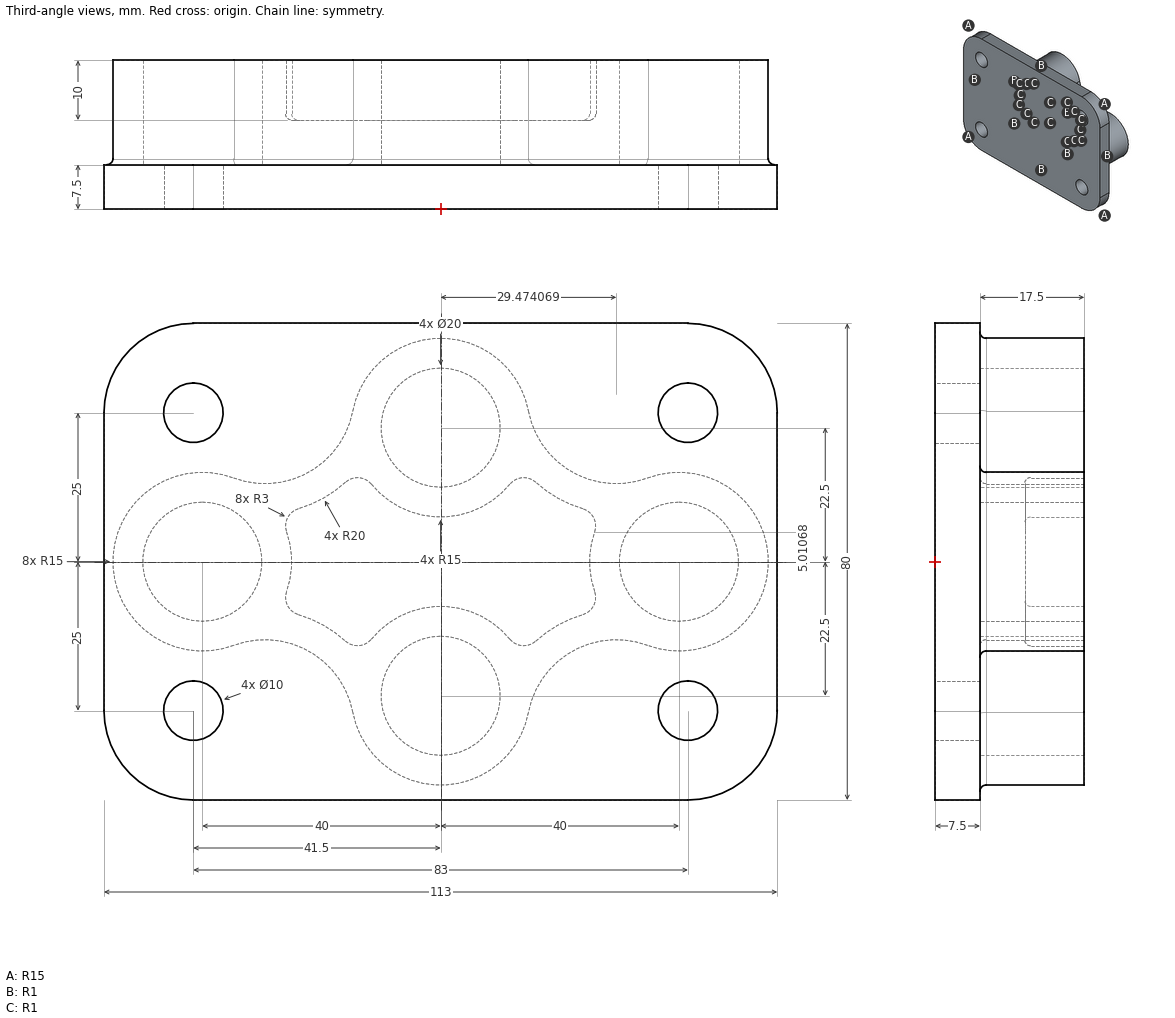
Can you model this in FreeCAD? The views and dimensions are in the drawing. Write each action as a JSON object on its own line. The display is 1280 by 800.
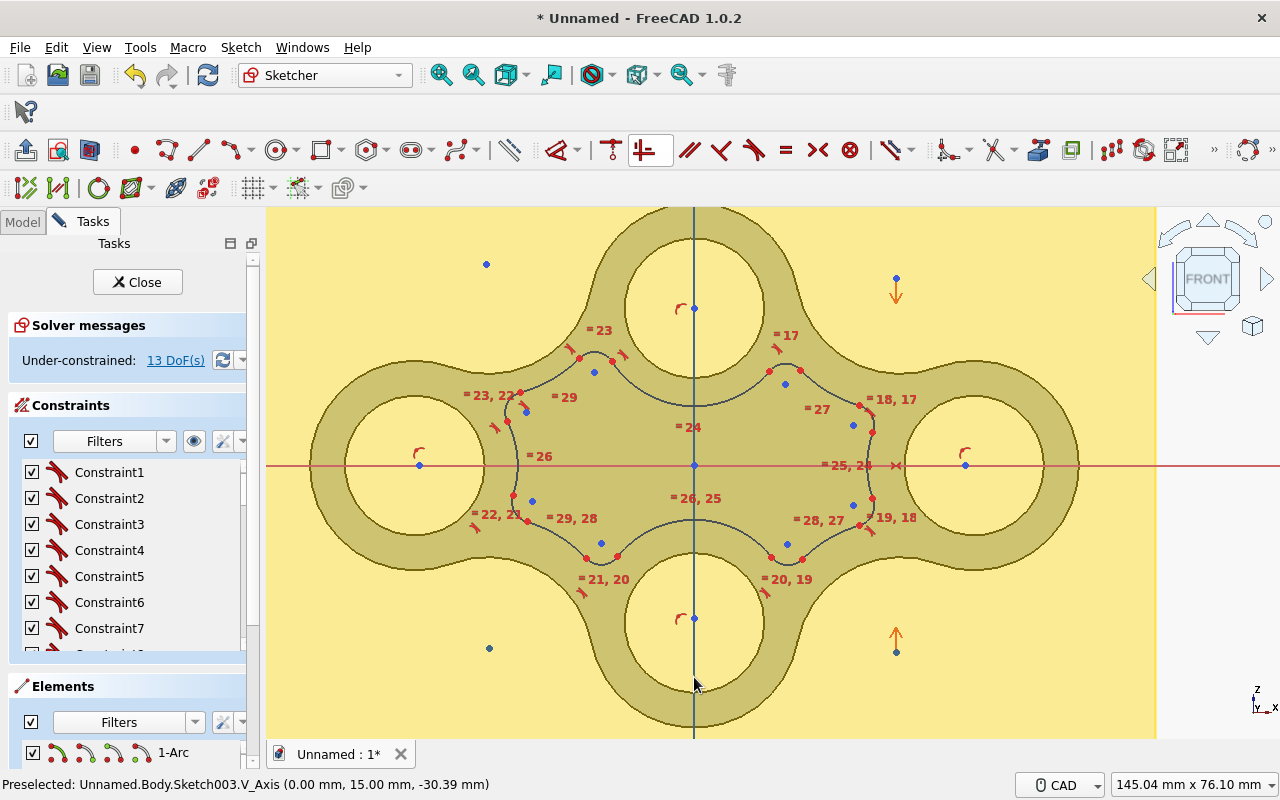
{"action": "key", "text": "s"}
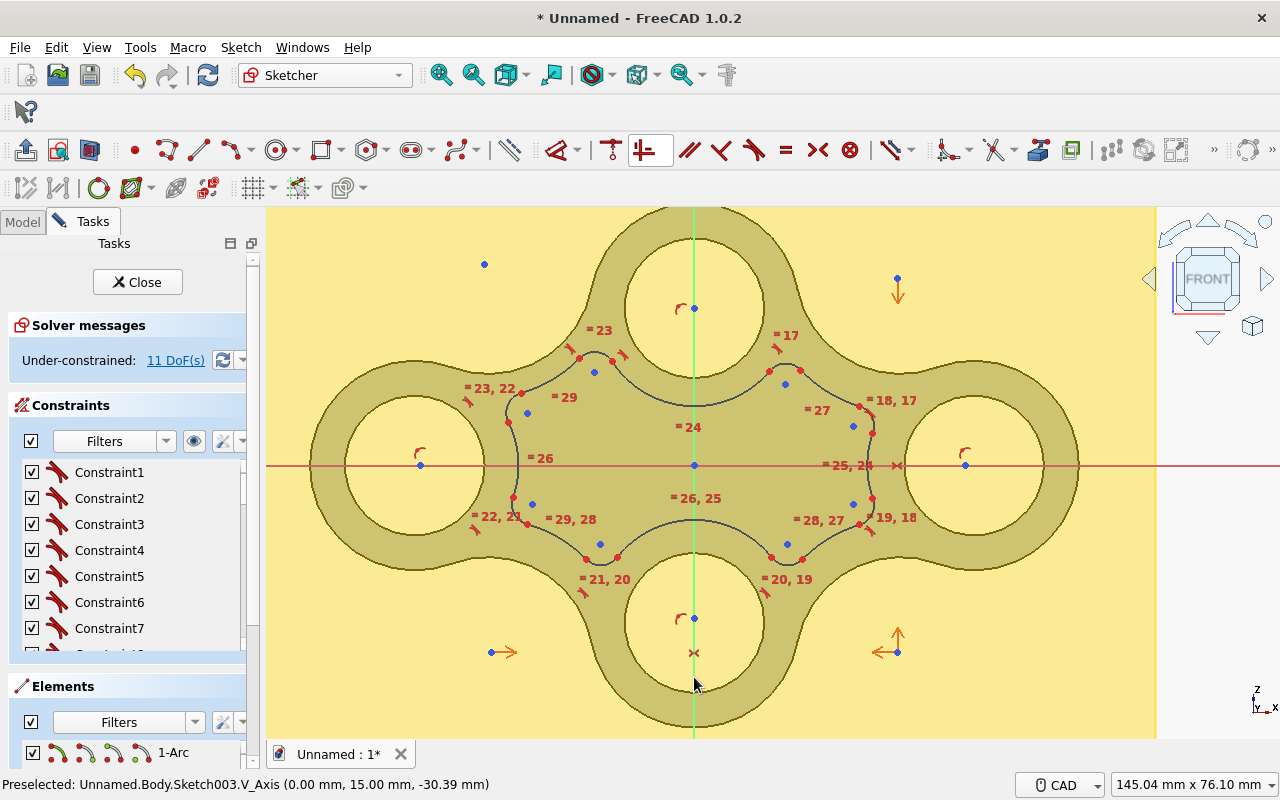
{"action": "left_click", "coordinate": [853, 426]}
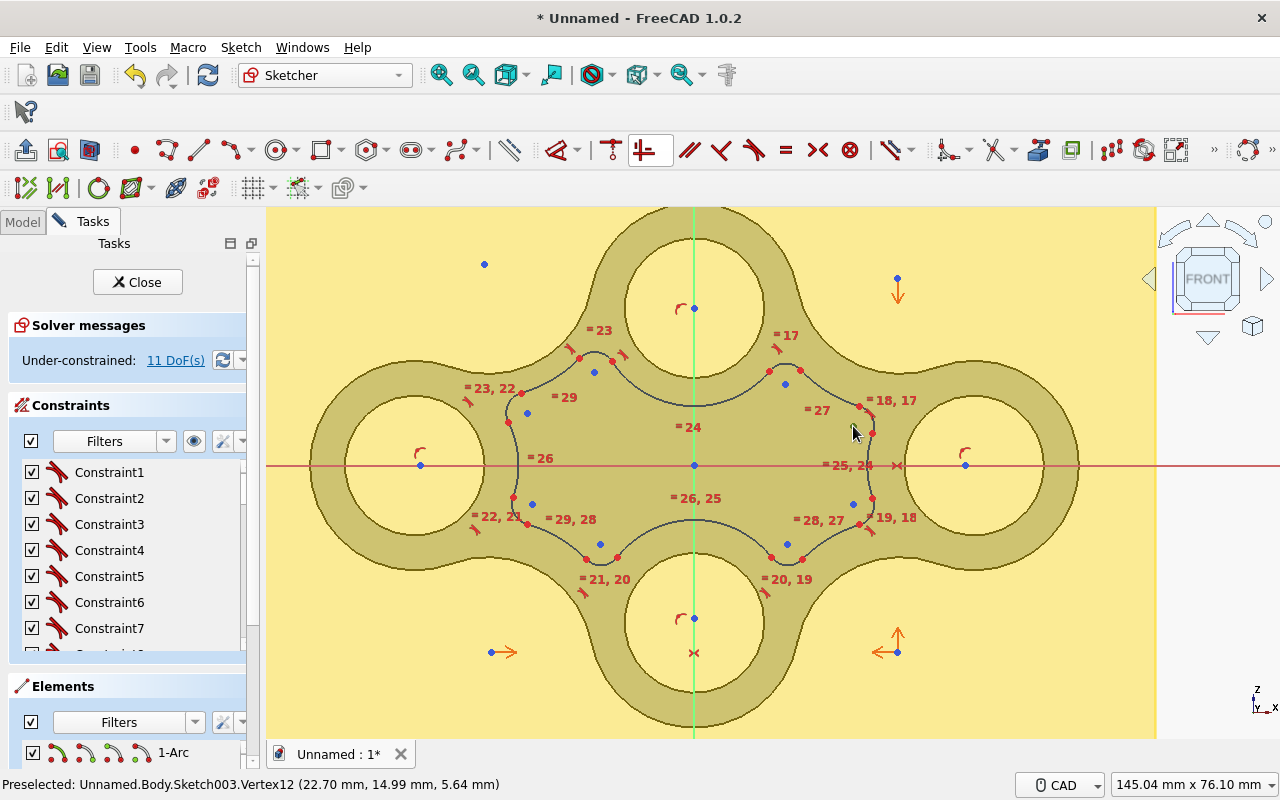
{"action": "left_click", "coordinate": [527, 413]}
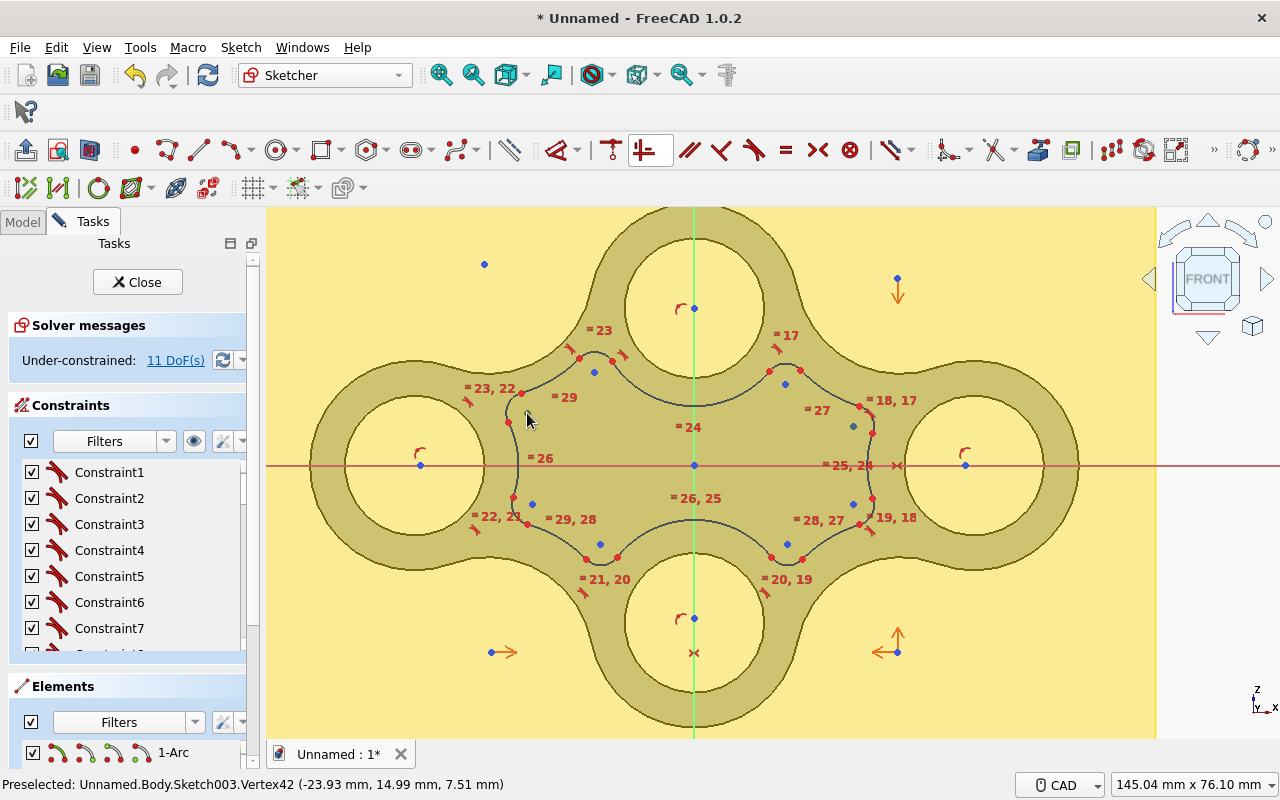
{"action": "left_click", "coordinate": [694, 677]}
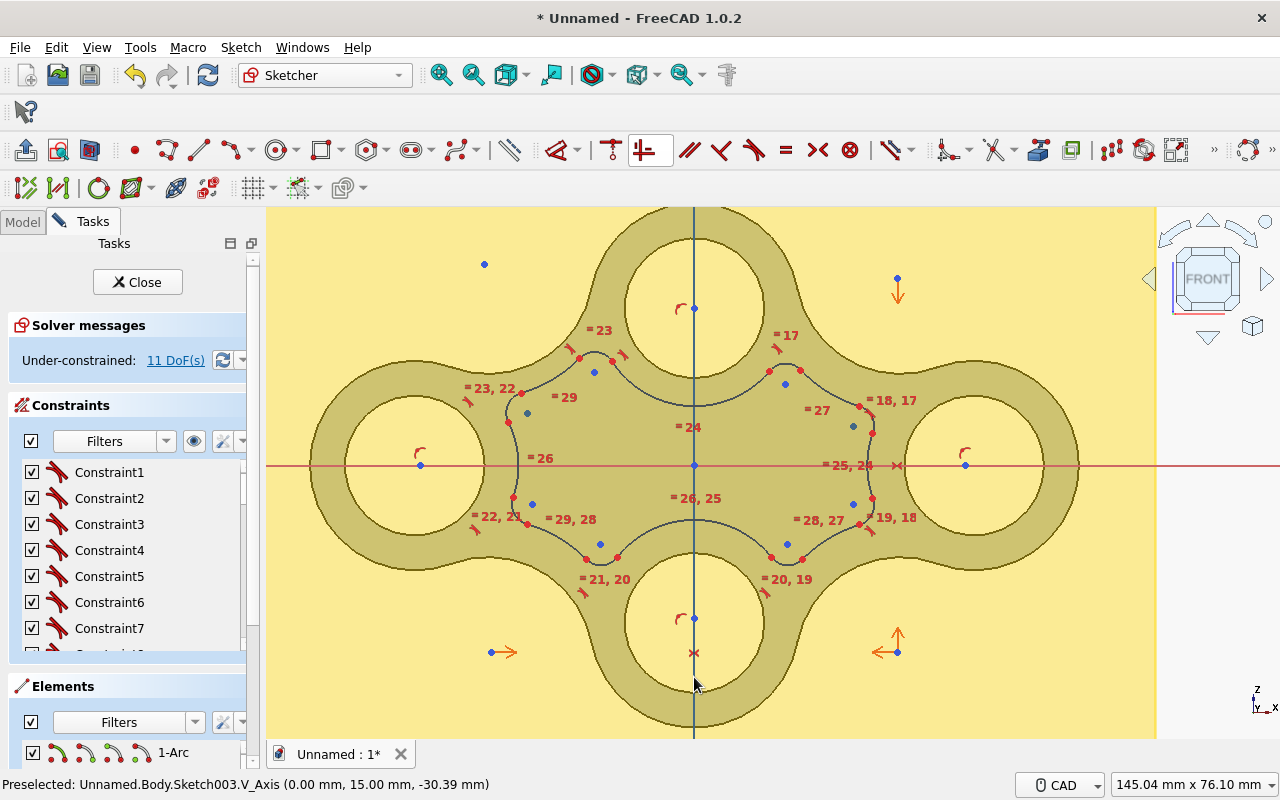
{"action": "key", "text": "s"}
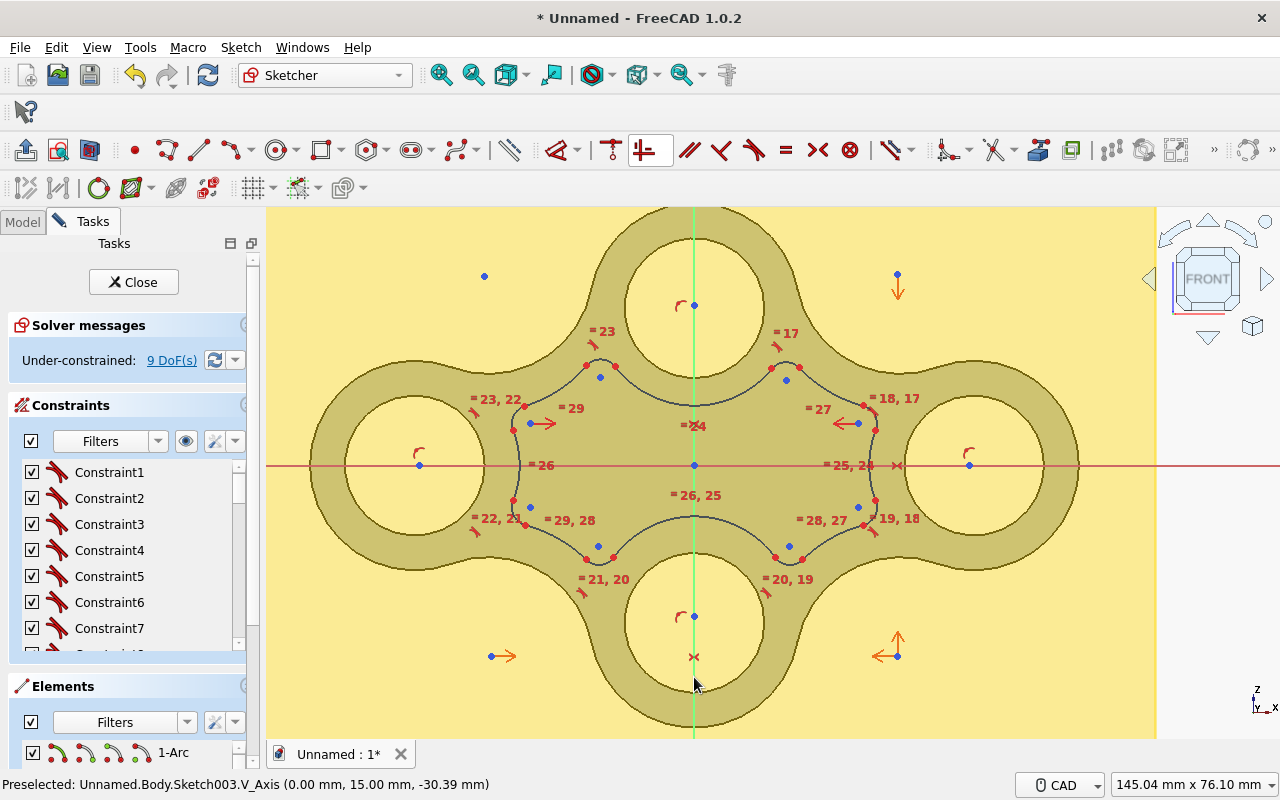
{"action": "left_click", "coordinate": [599, 547]}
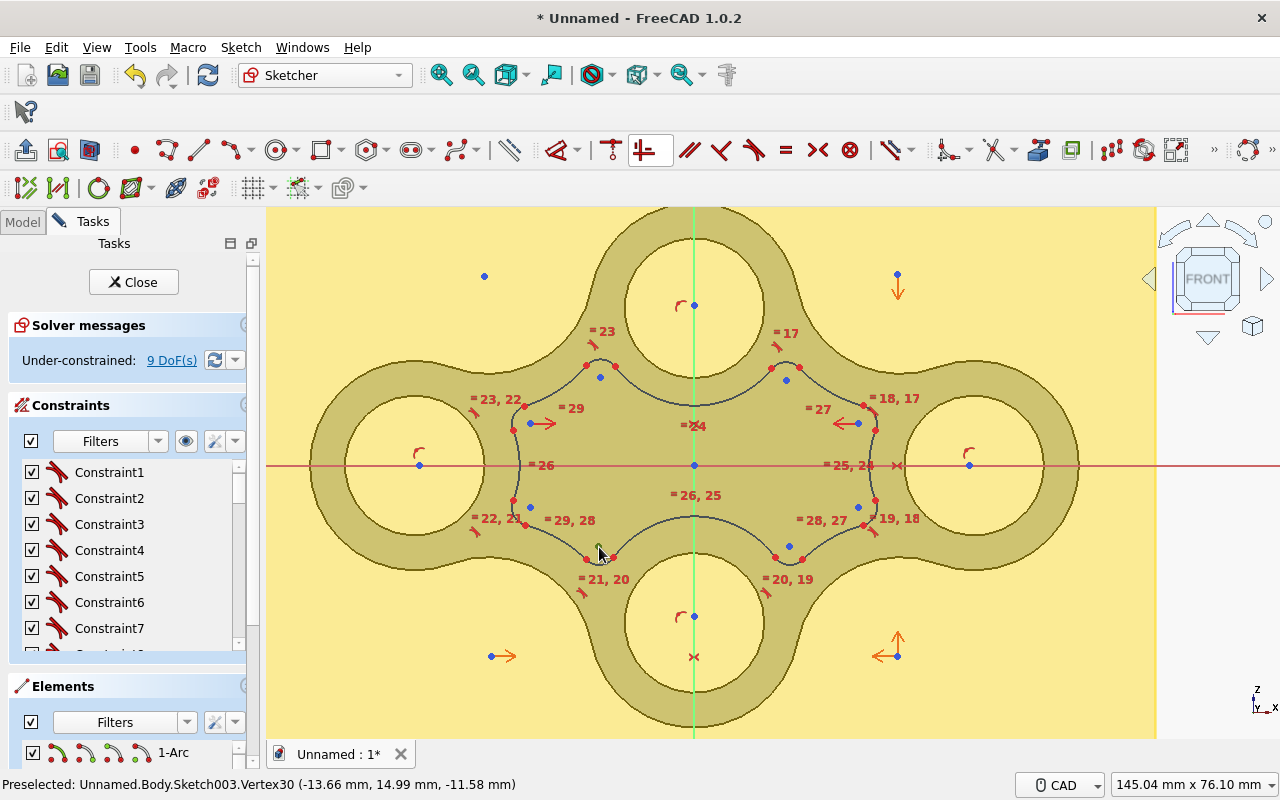
{"action": "left_click", "coordinate": [601, 378]}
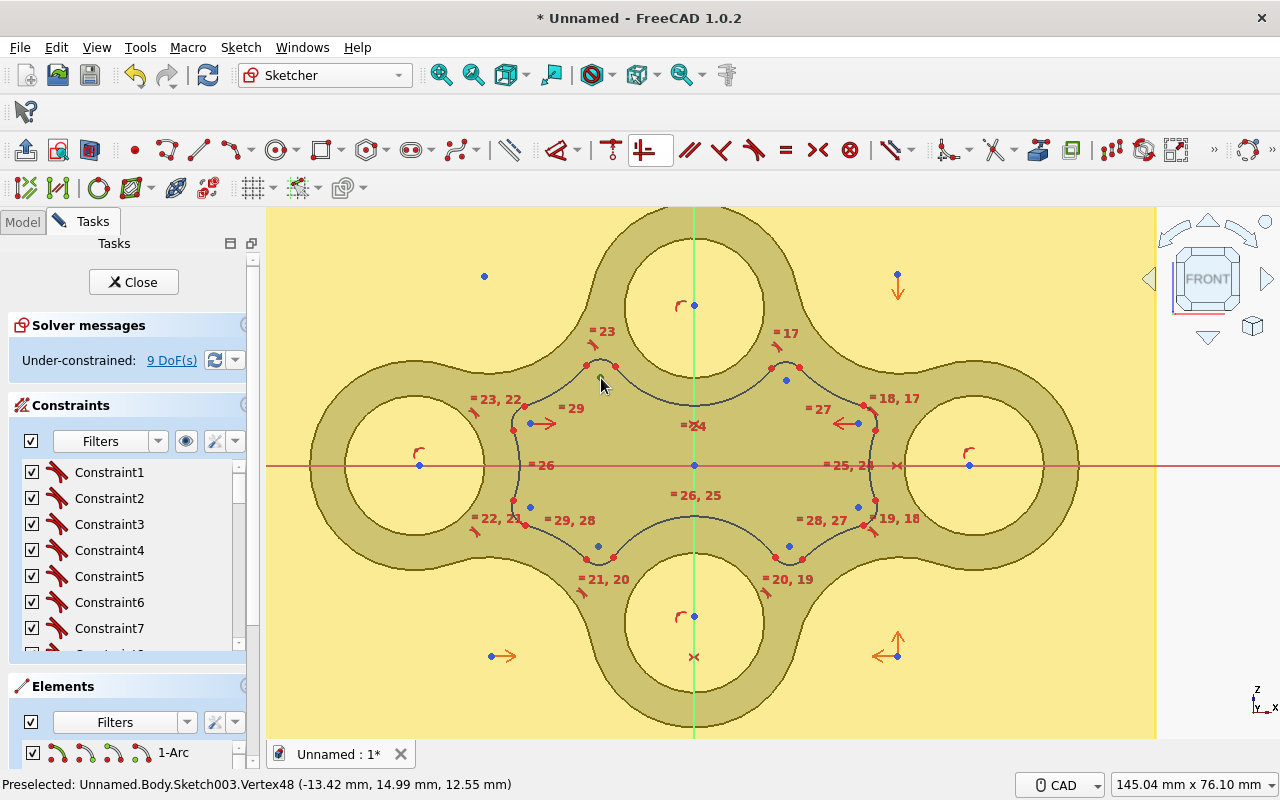
{"action": "left_click", "coordinate": [353, 466]}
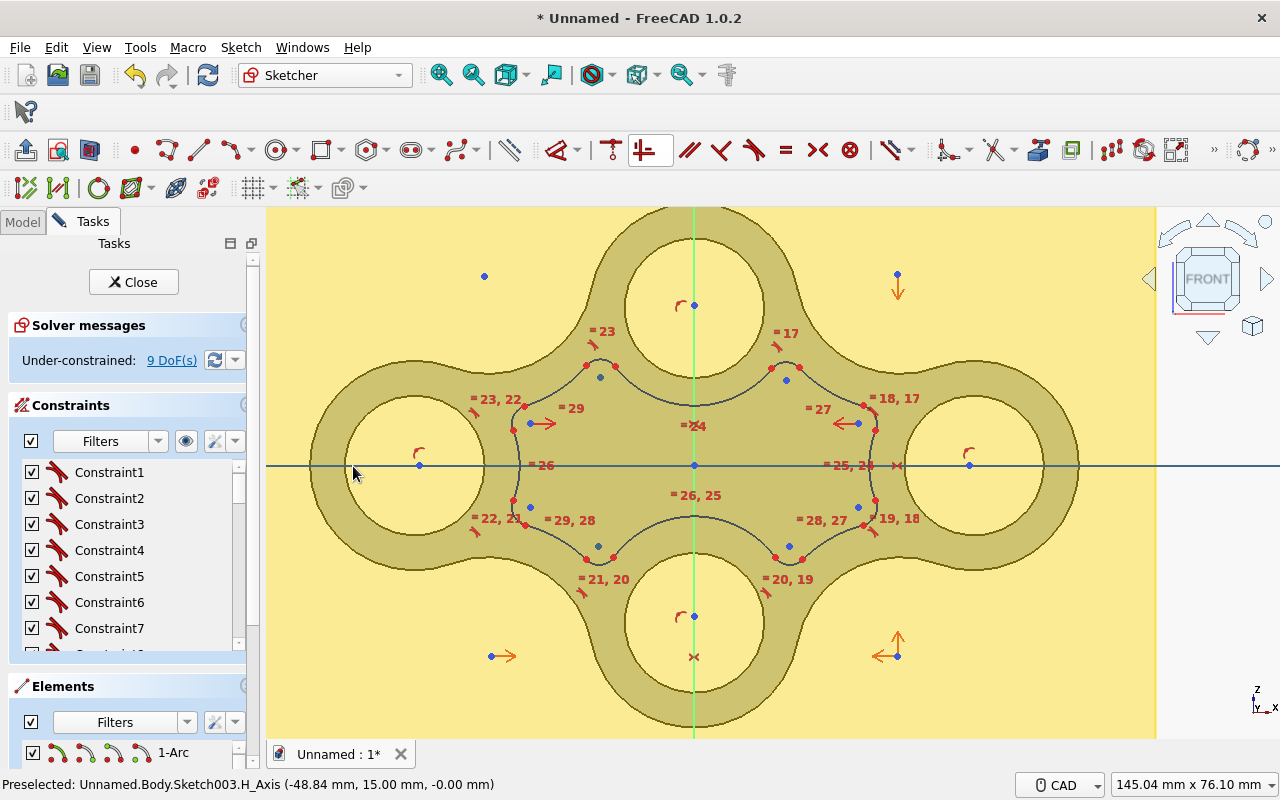
{"action": "key", "text": "s"}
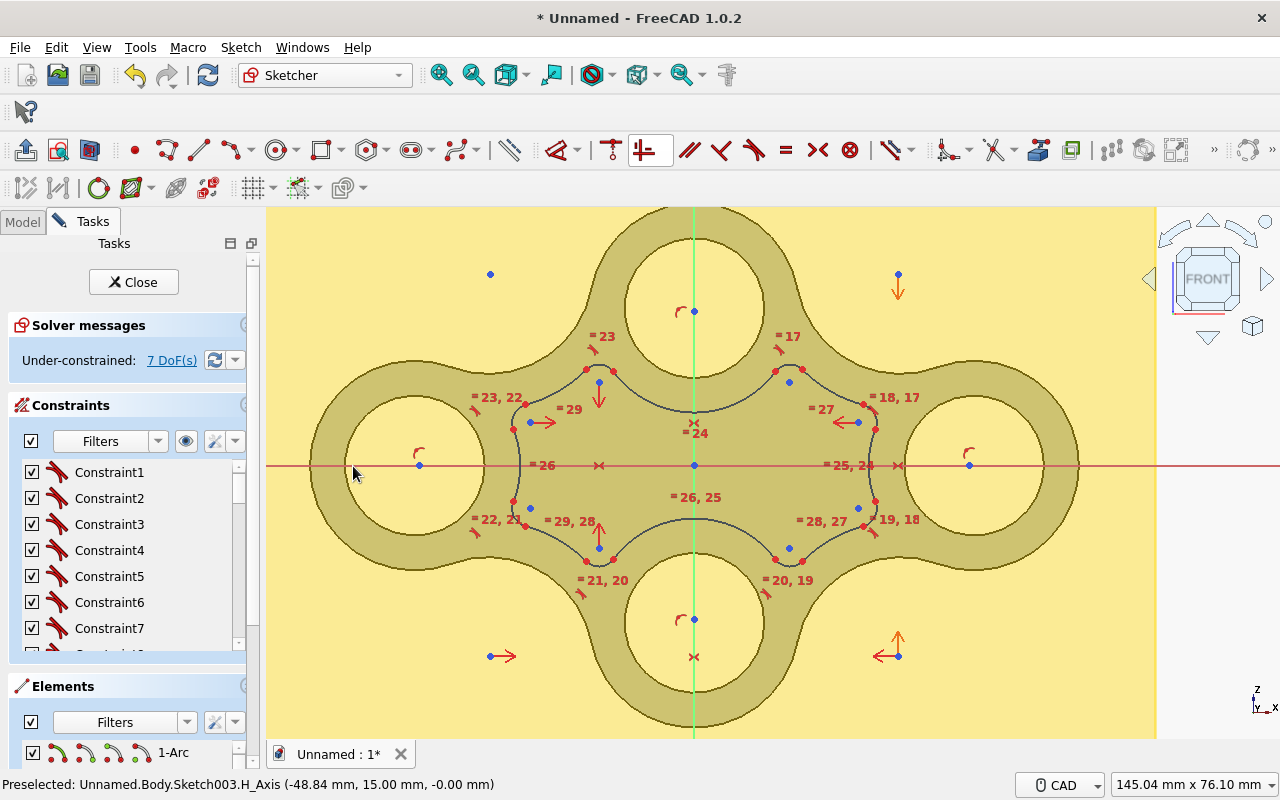
{"action": "key", "text": "d"}